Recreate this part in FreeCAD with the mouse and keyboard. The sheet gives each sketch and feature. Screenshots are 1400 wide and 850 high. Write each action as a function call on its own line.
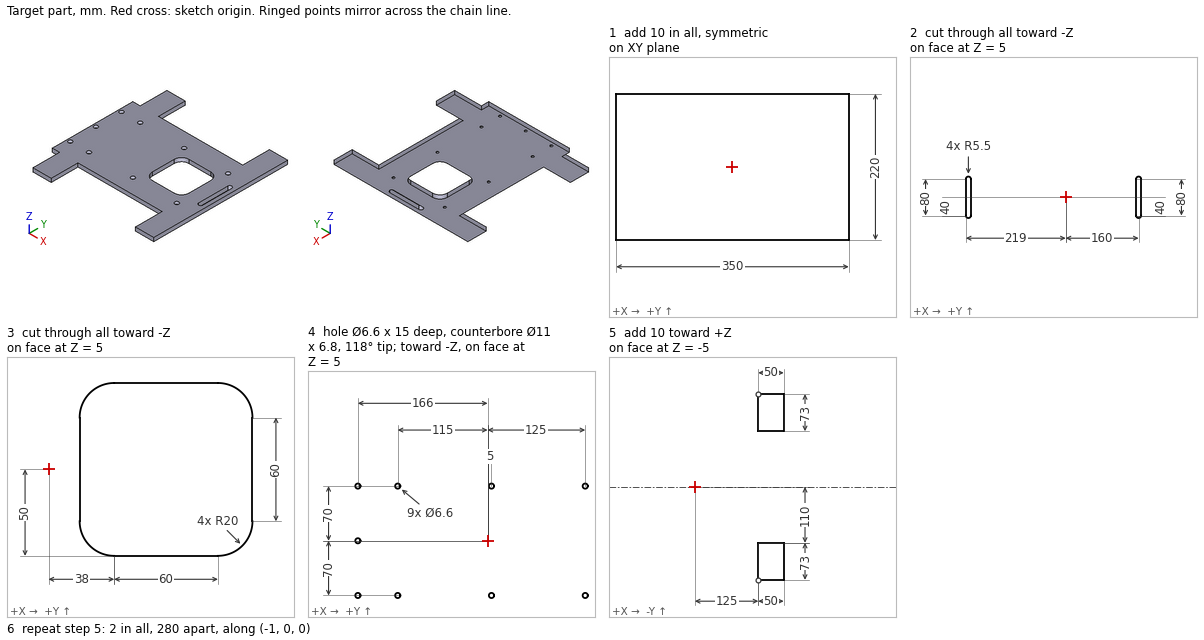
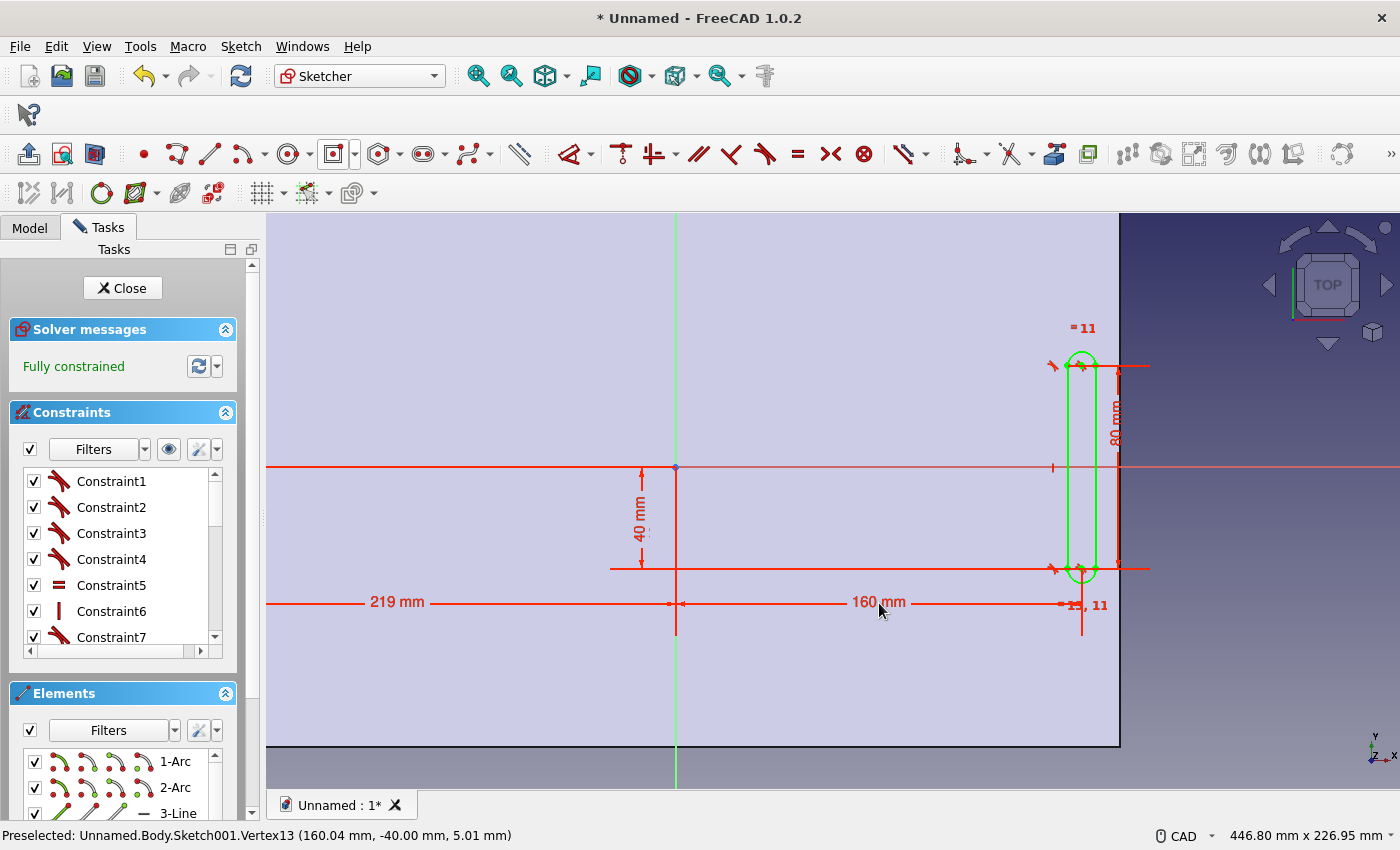
click(123, 288)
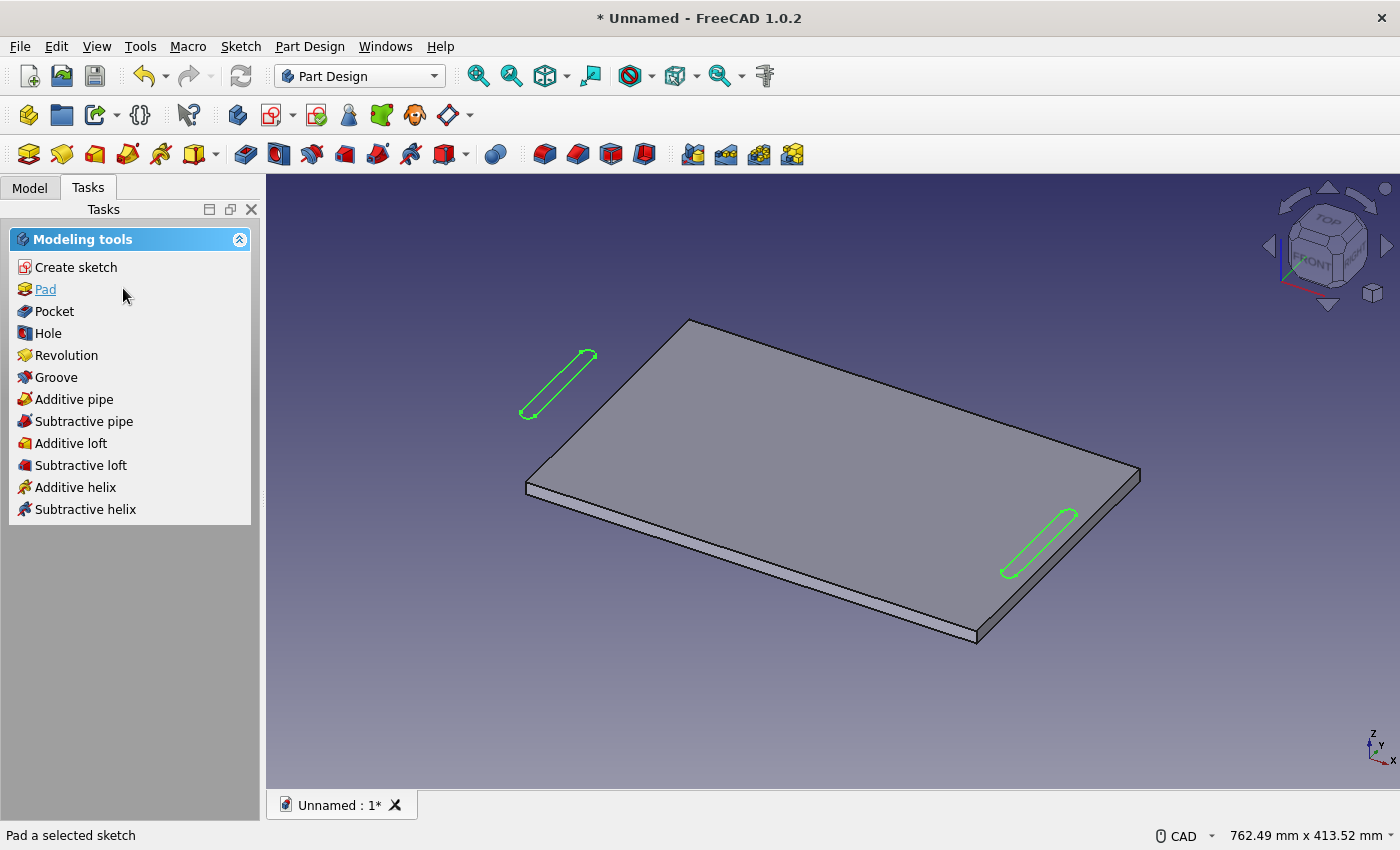
click(246, 154)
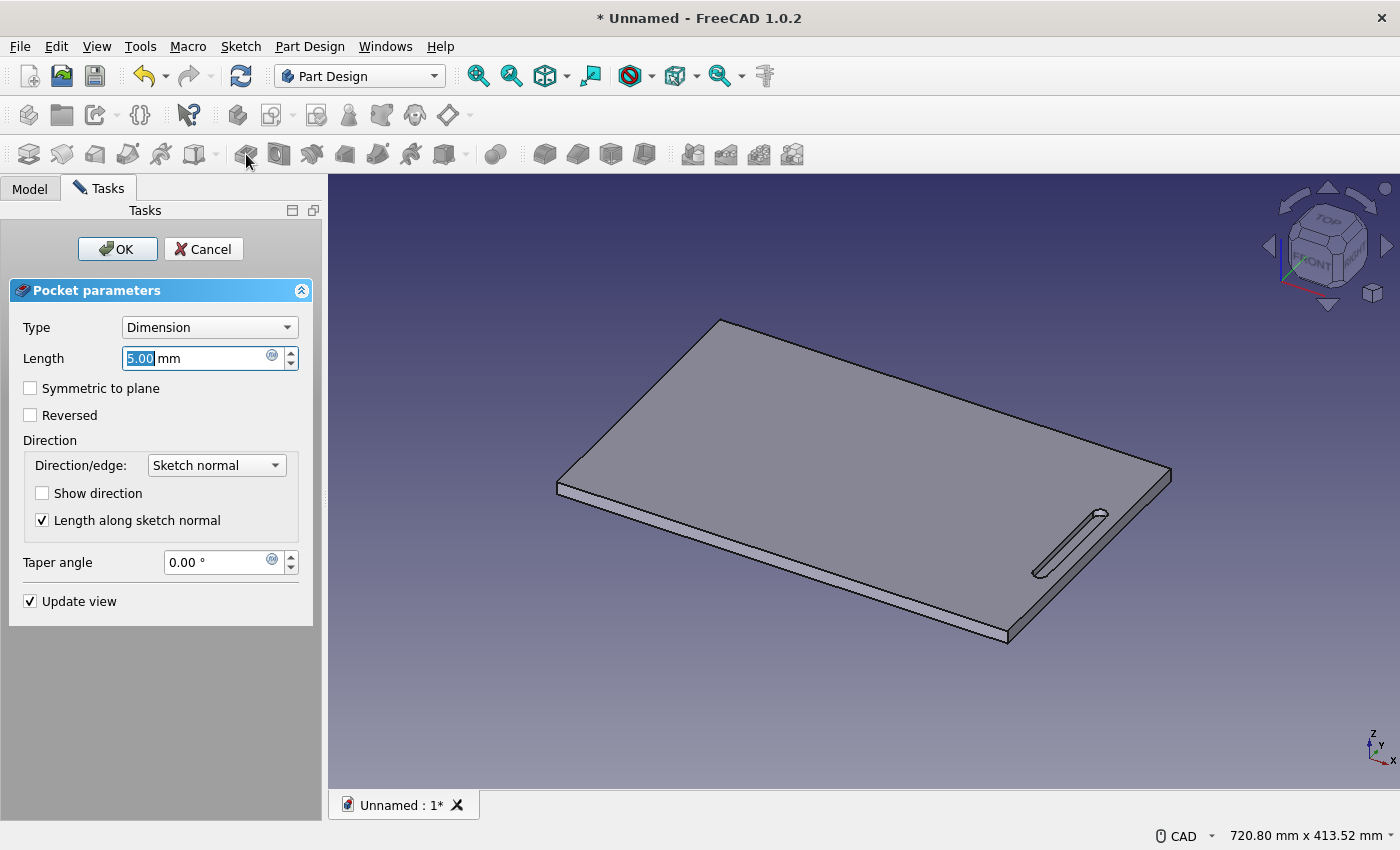
click(210, 328)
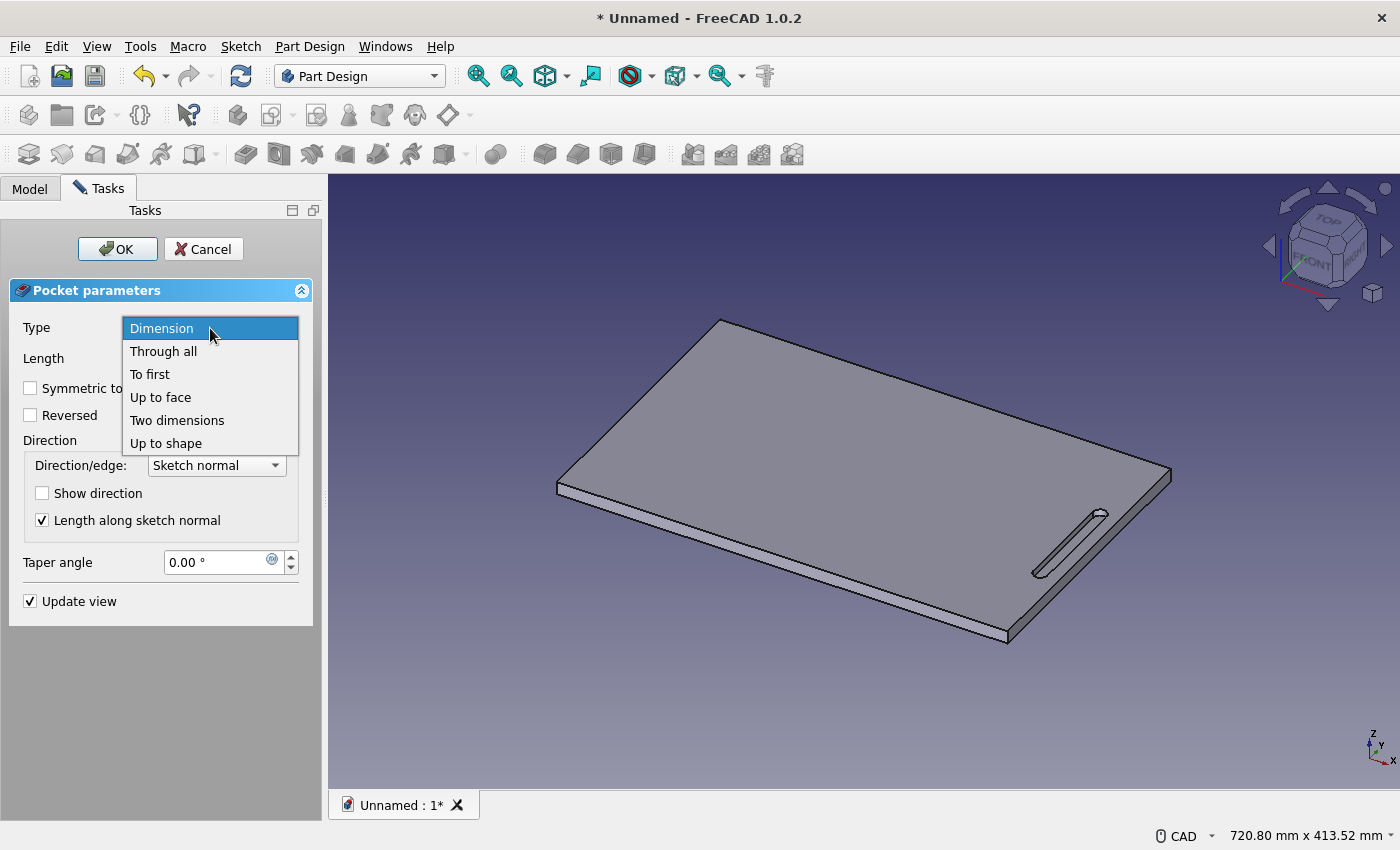
click(208, 352)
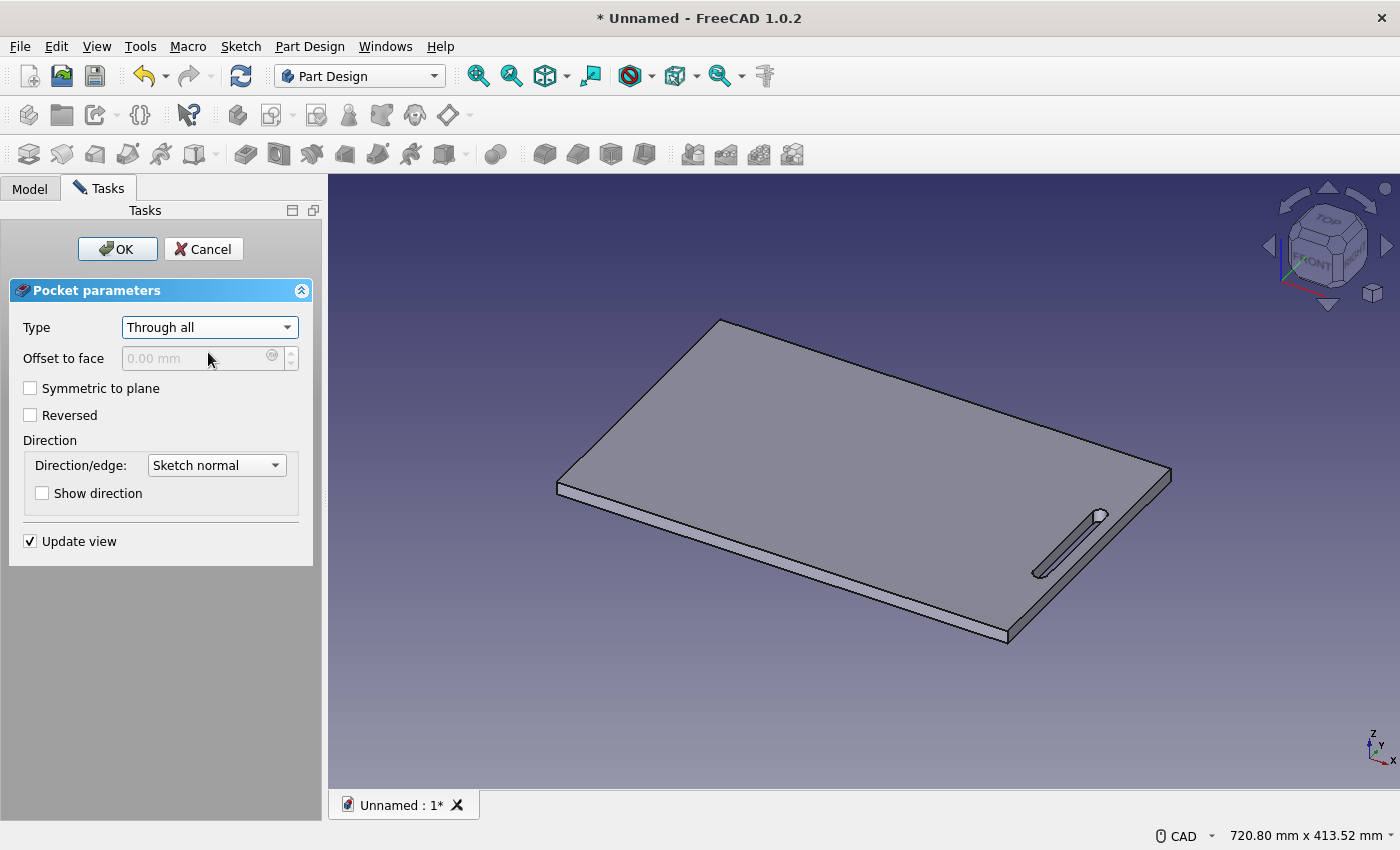
click(118, 249)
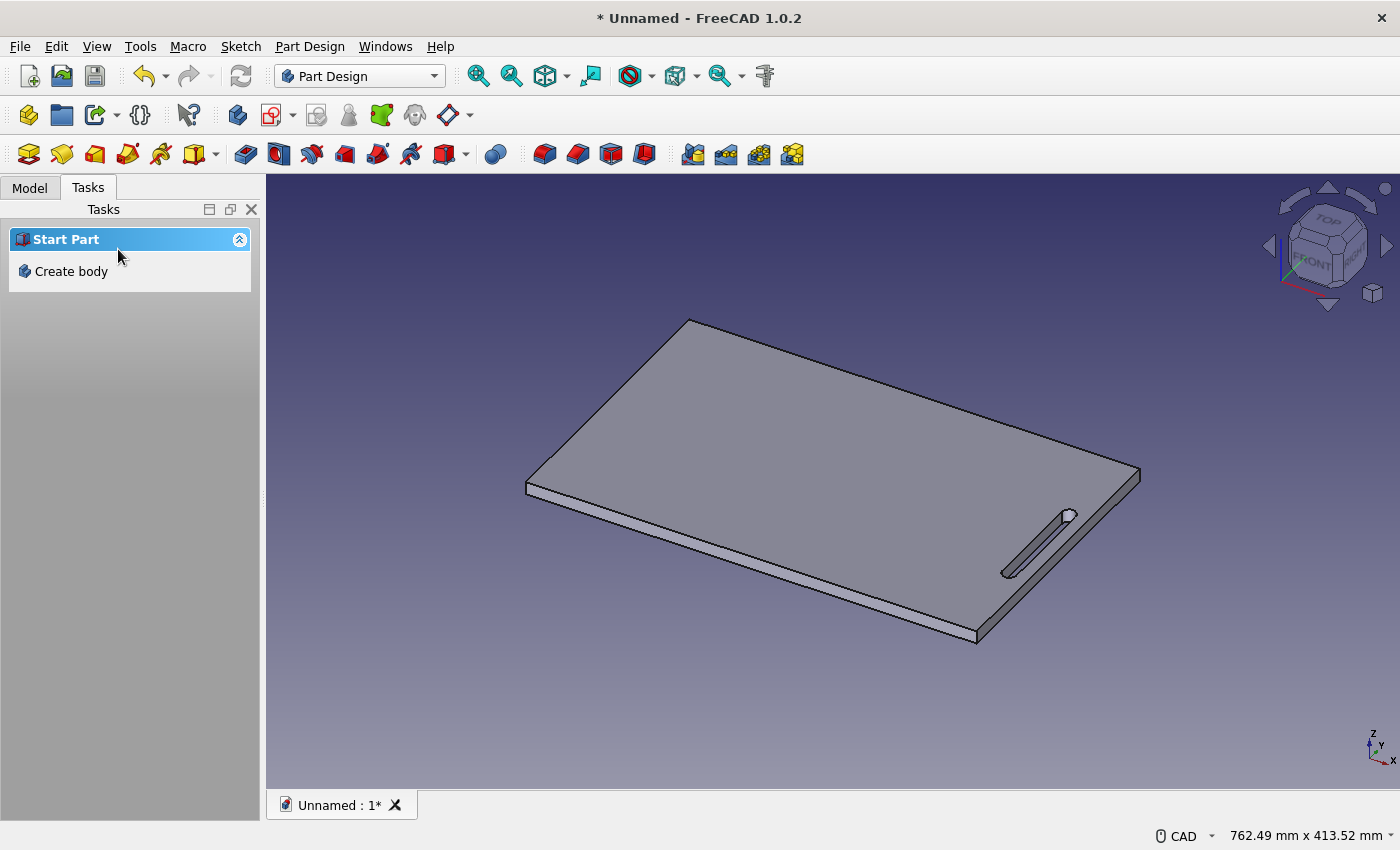
click(833, 474)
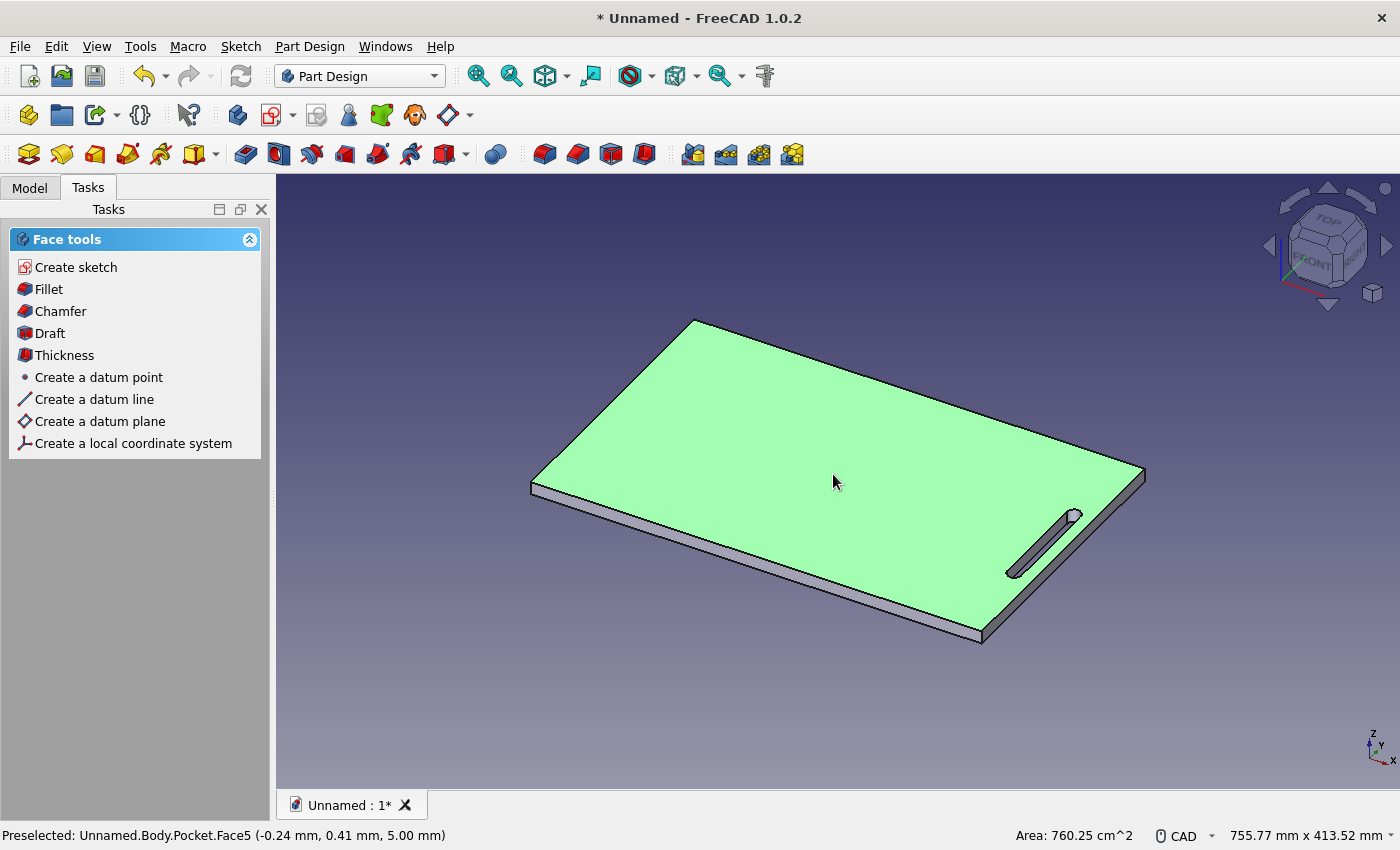
click(270, 116)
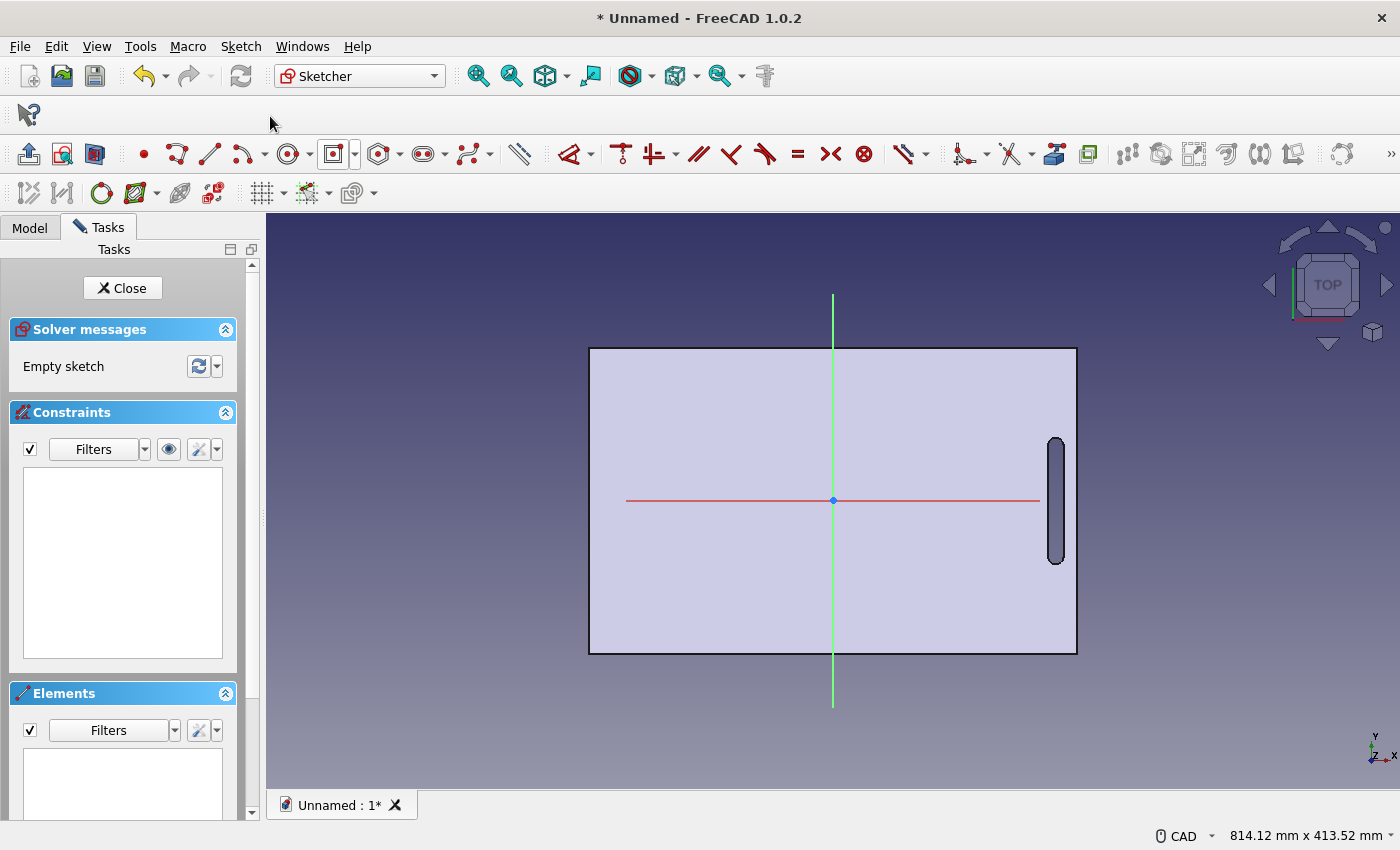
scroll(1003, 501, up, 5)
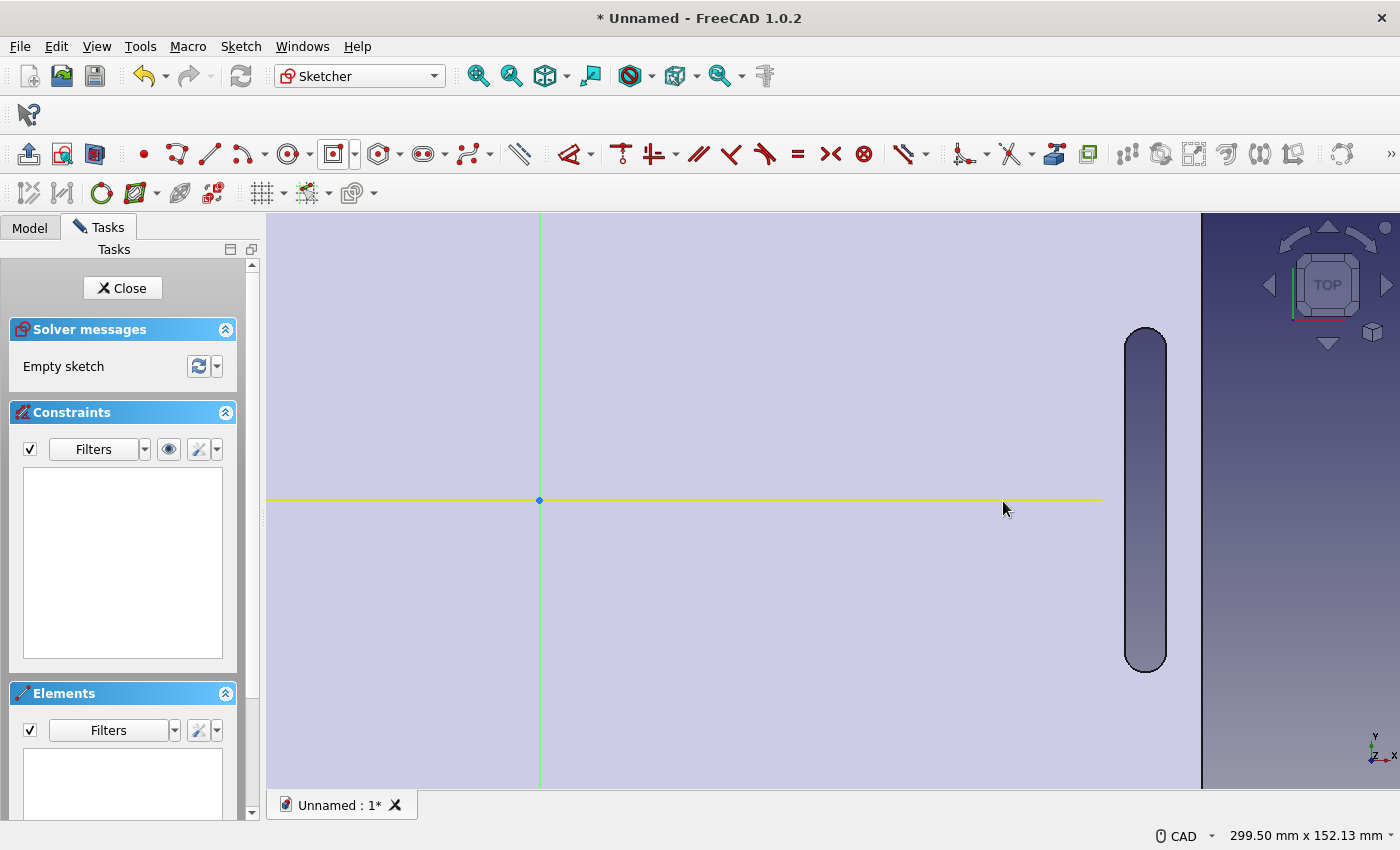
key(g)
key(l)